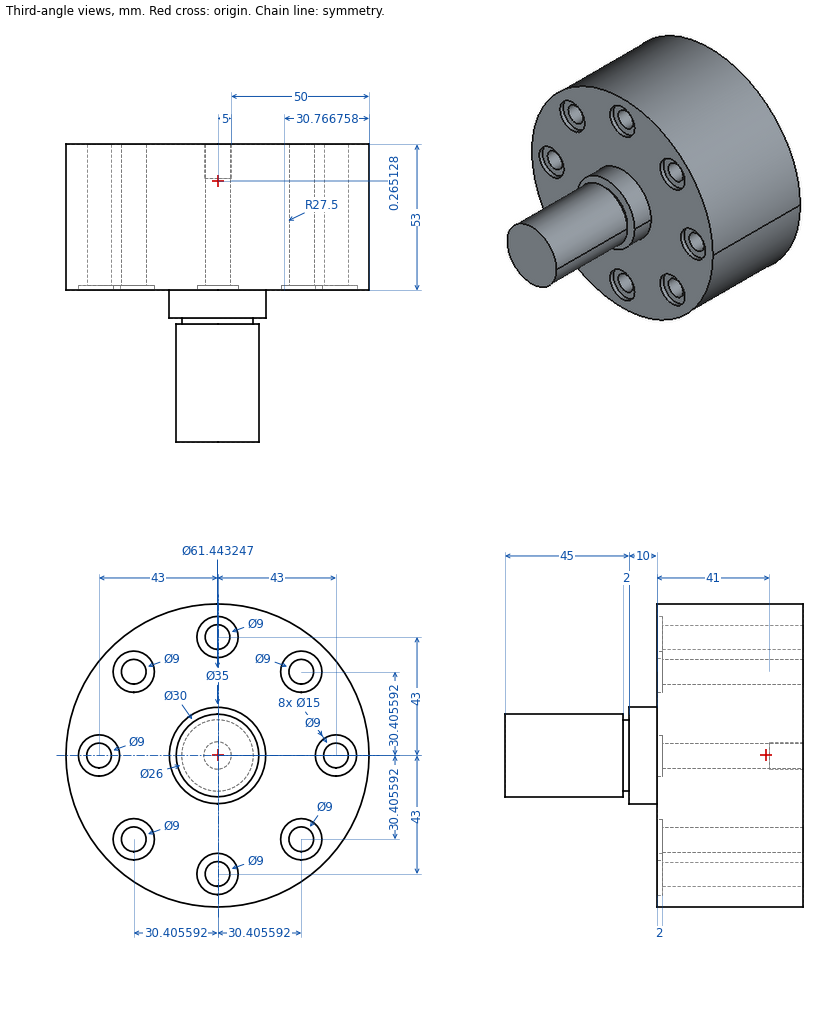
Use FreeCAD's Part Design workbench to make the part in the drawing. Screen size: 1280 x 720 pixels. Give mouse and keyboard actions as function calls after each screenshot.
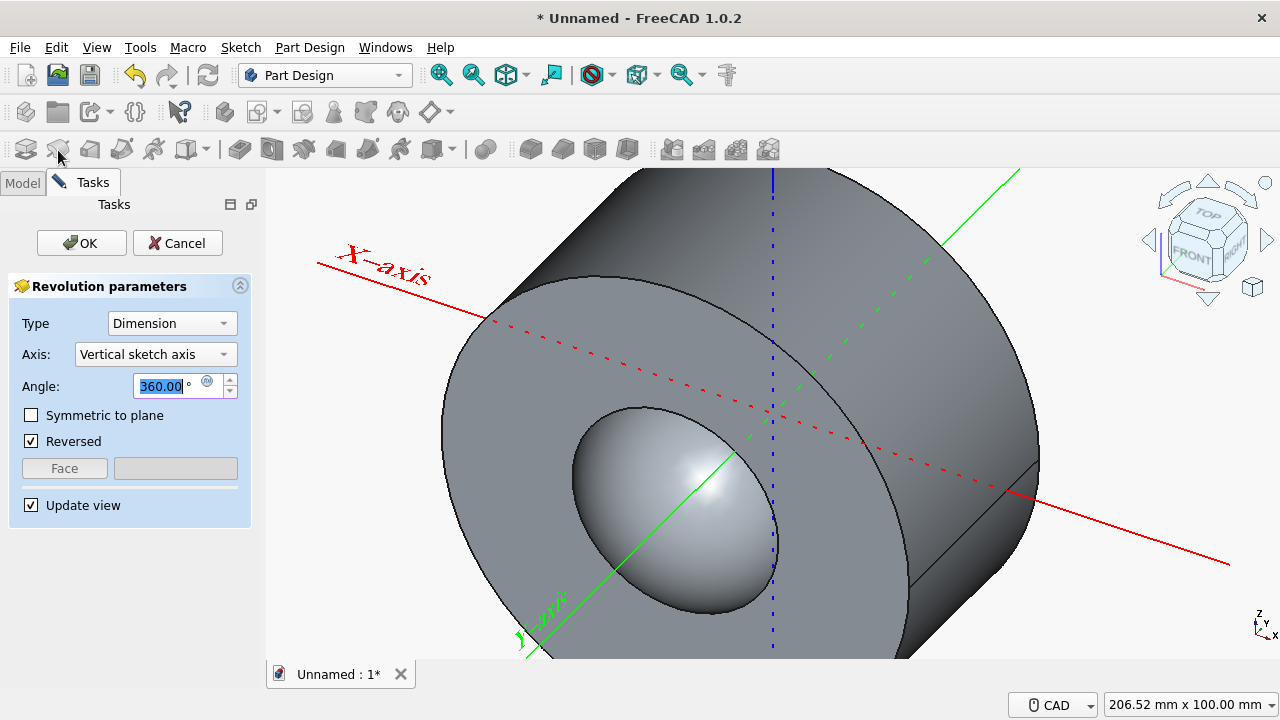
click(82, 243)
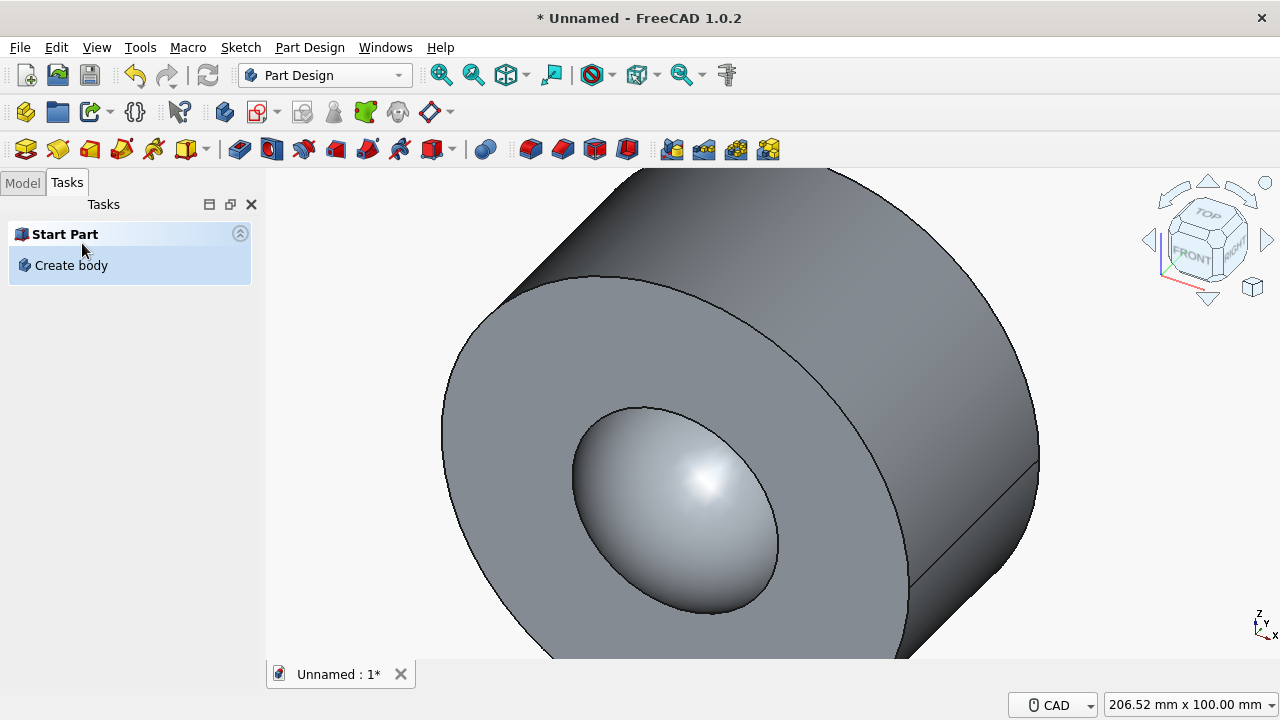
click(442, 76)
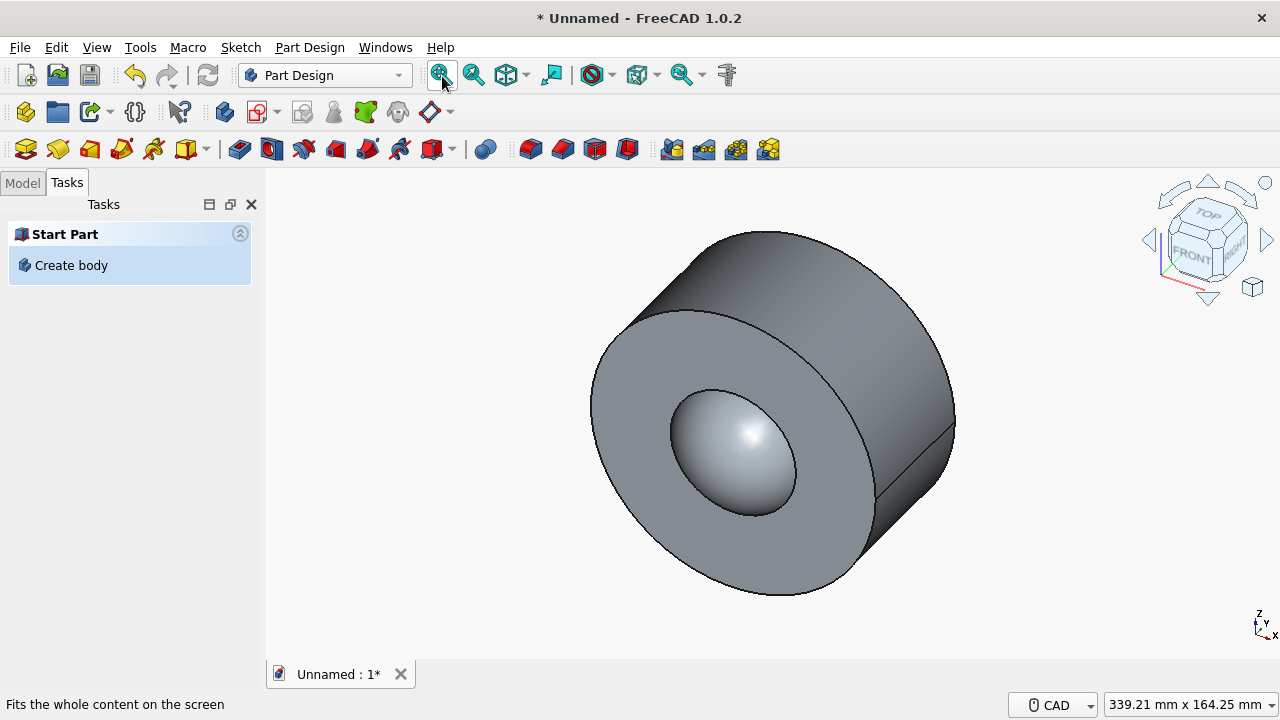
click(774, 388)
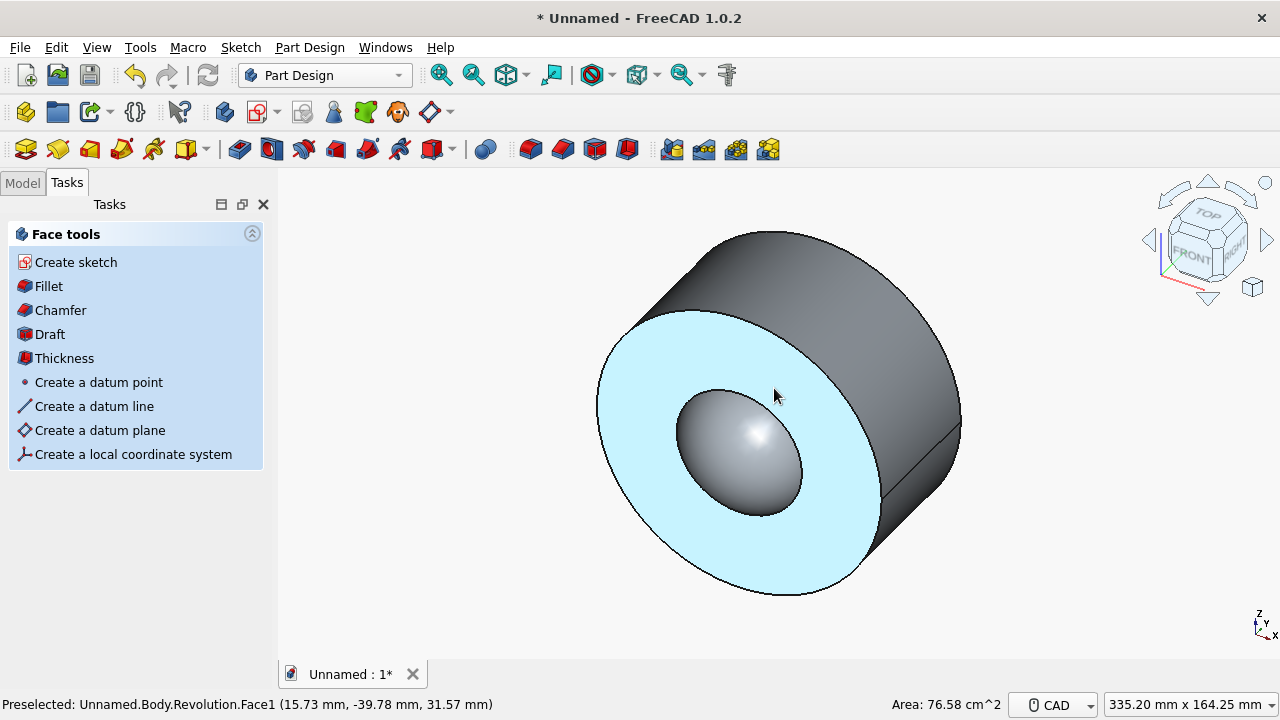
click(258, 112)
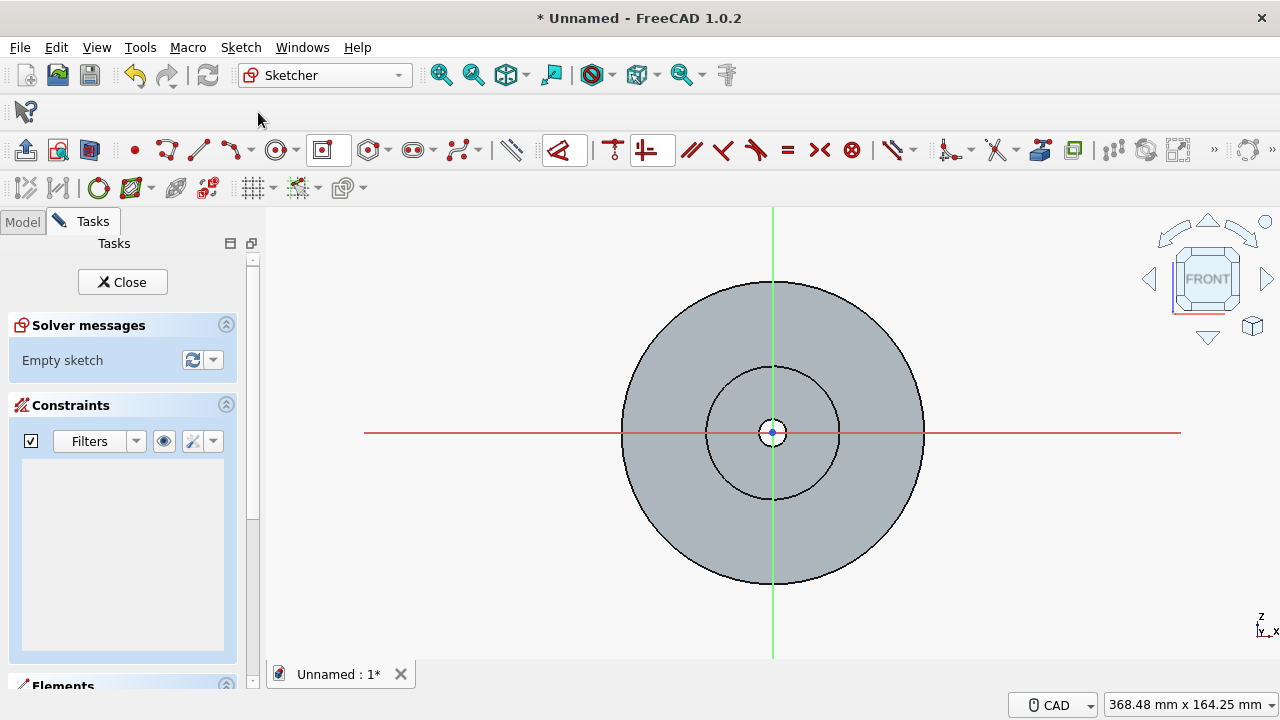
key(g)
key(c)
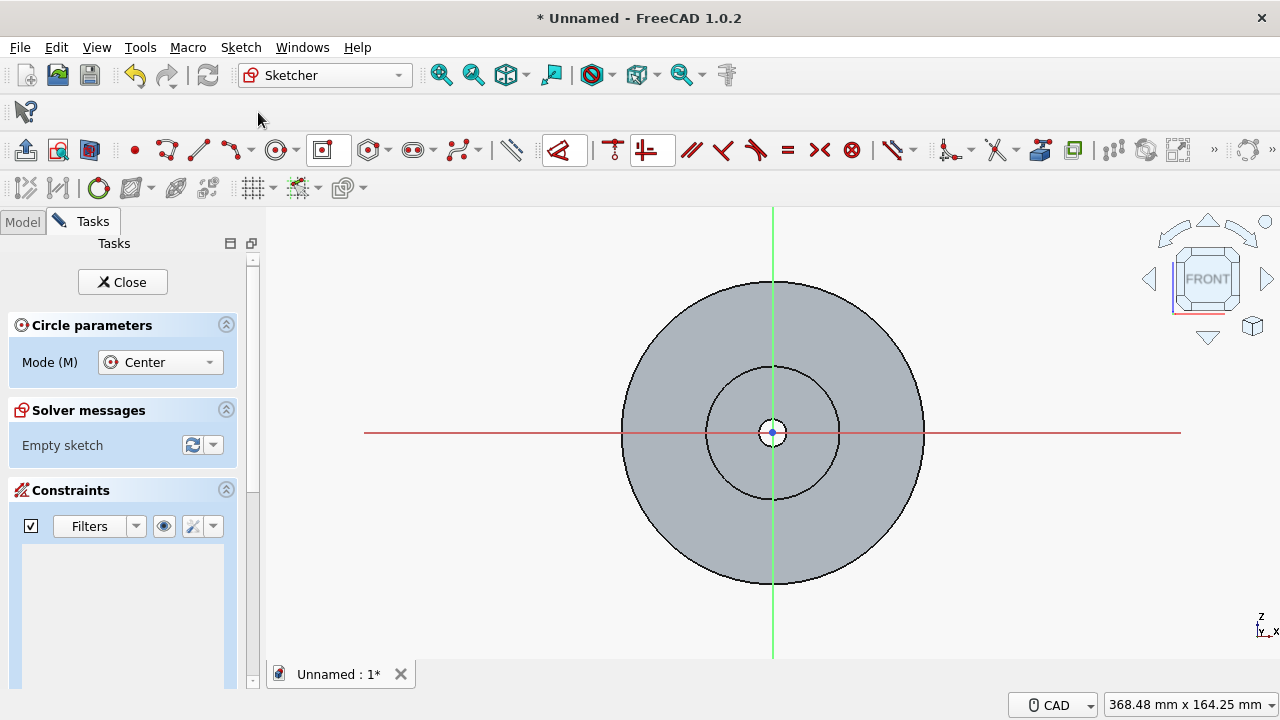
click(891, 433)
move(906, 418)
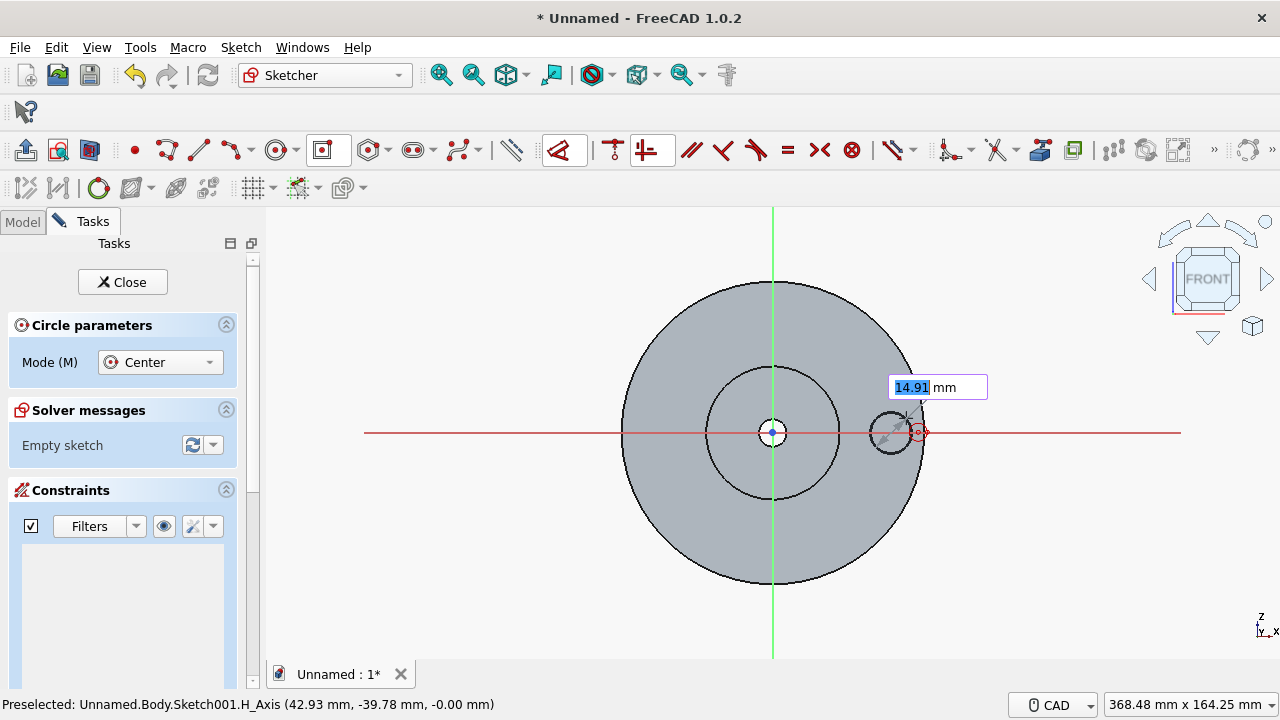
text(15)
key(Return)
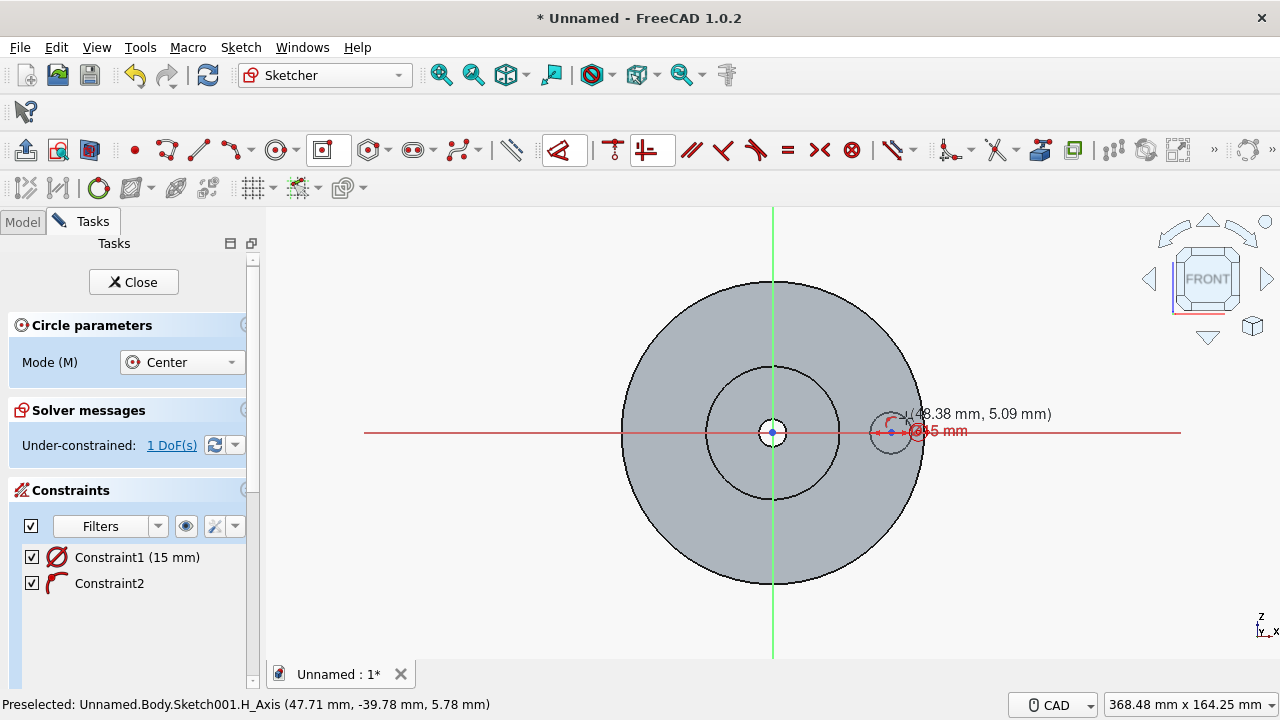
click(857, 517)
move(871, 502)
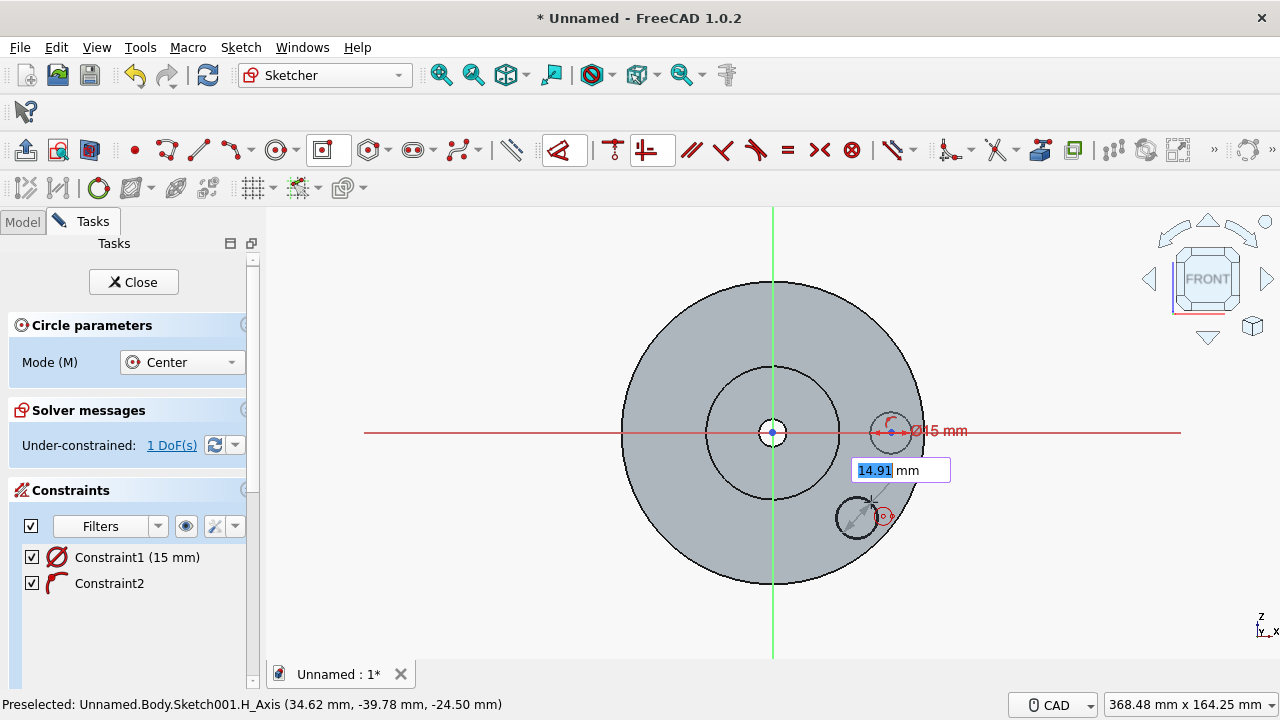
text(15)
key(Return)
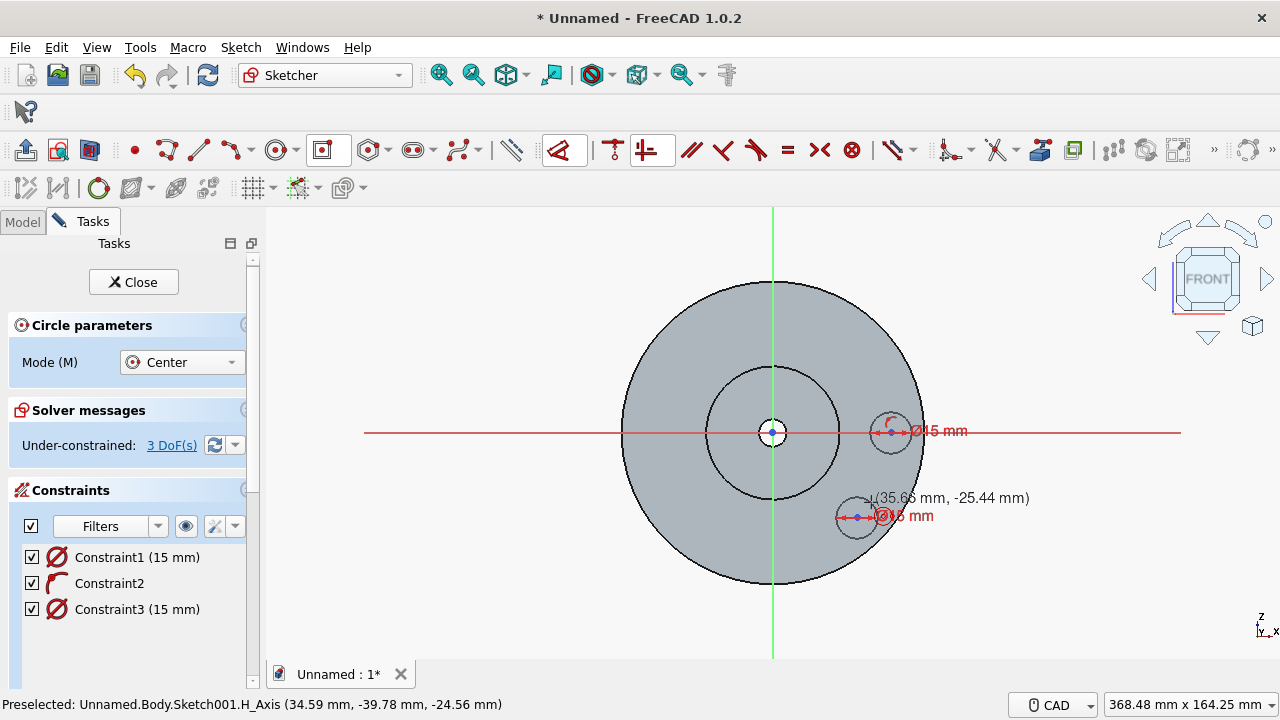
click(773, 551)
move(787, 537)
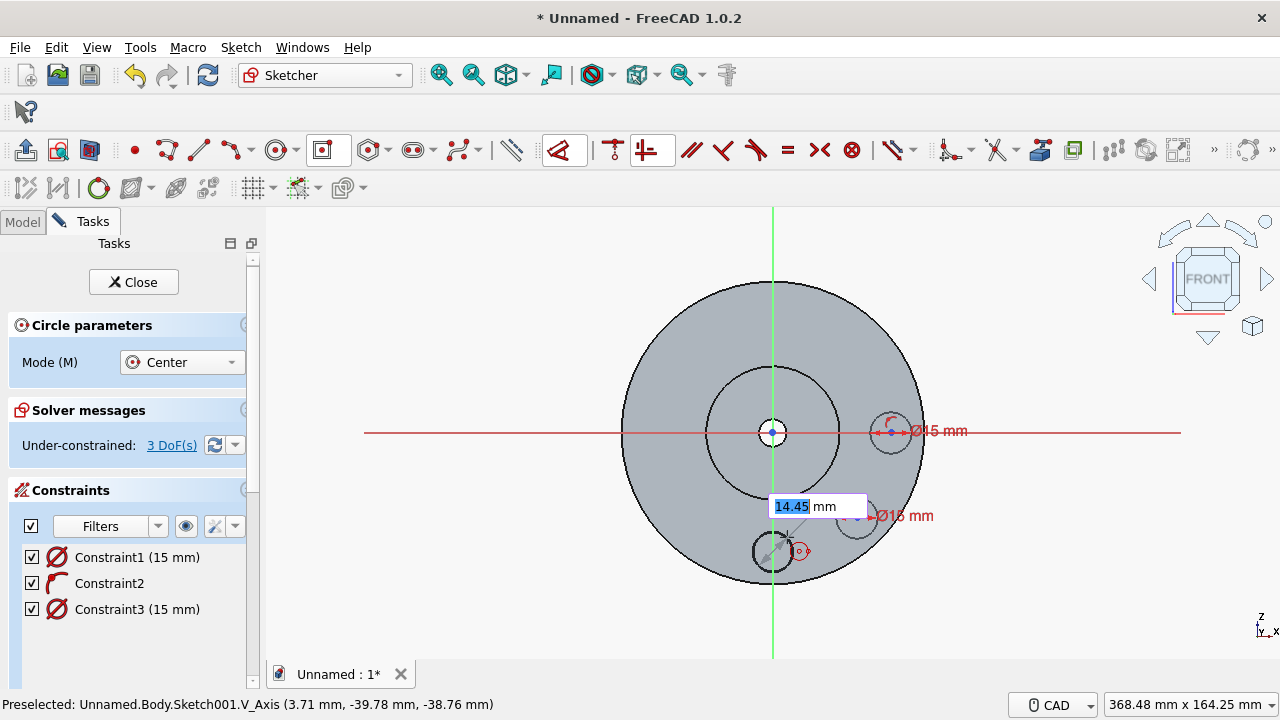
text(15)
key(Return)